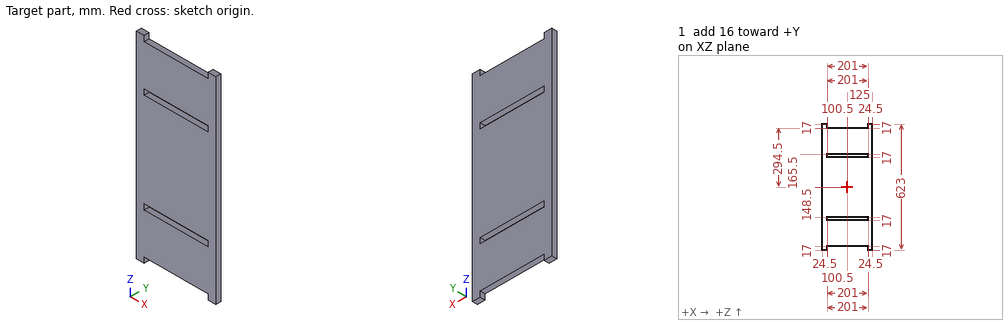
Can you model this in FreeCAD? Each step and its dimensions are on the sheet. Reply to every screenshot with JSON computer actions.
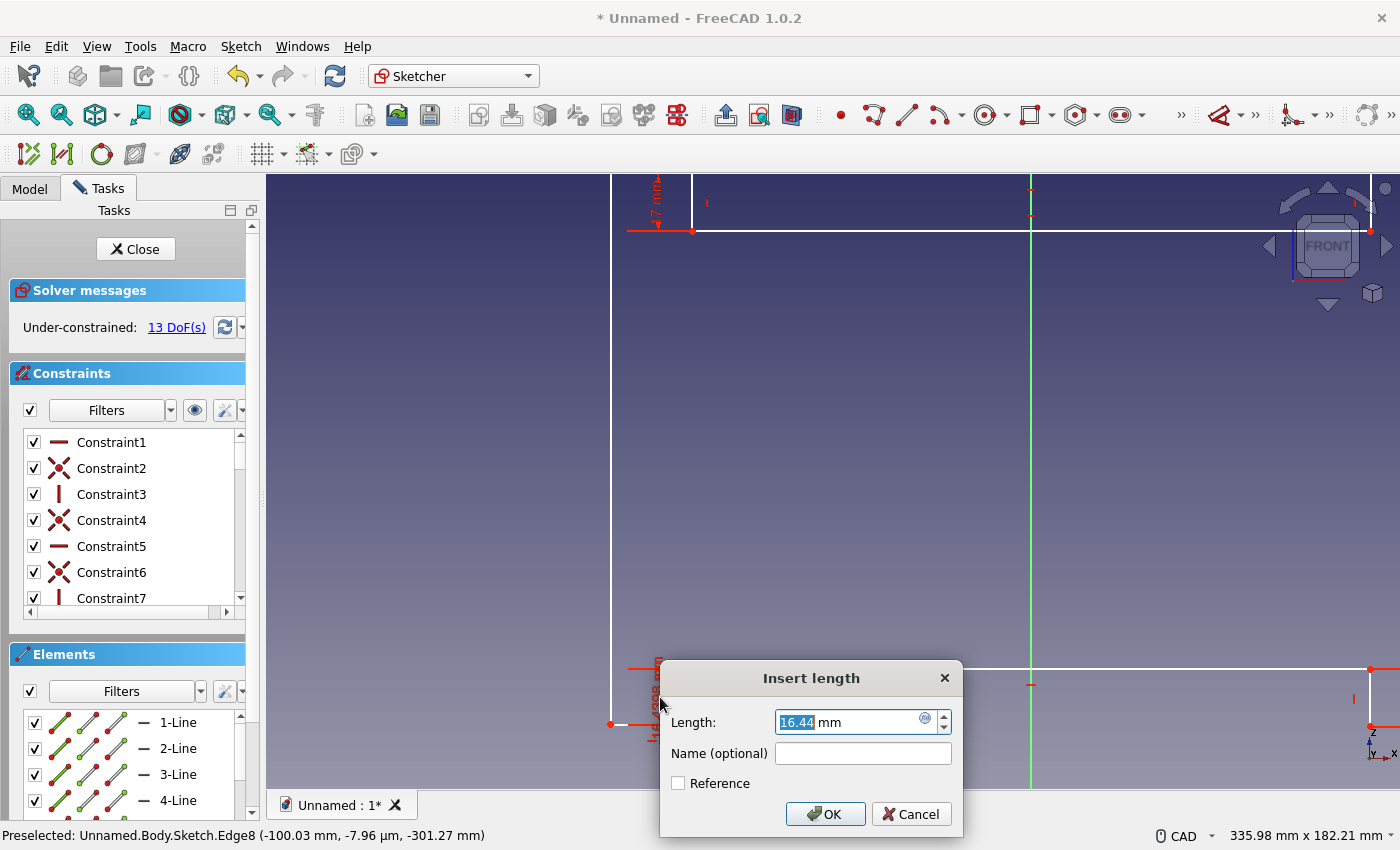
{"action": "type", "text": "17"}
{"action": "key", "text": "Return"}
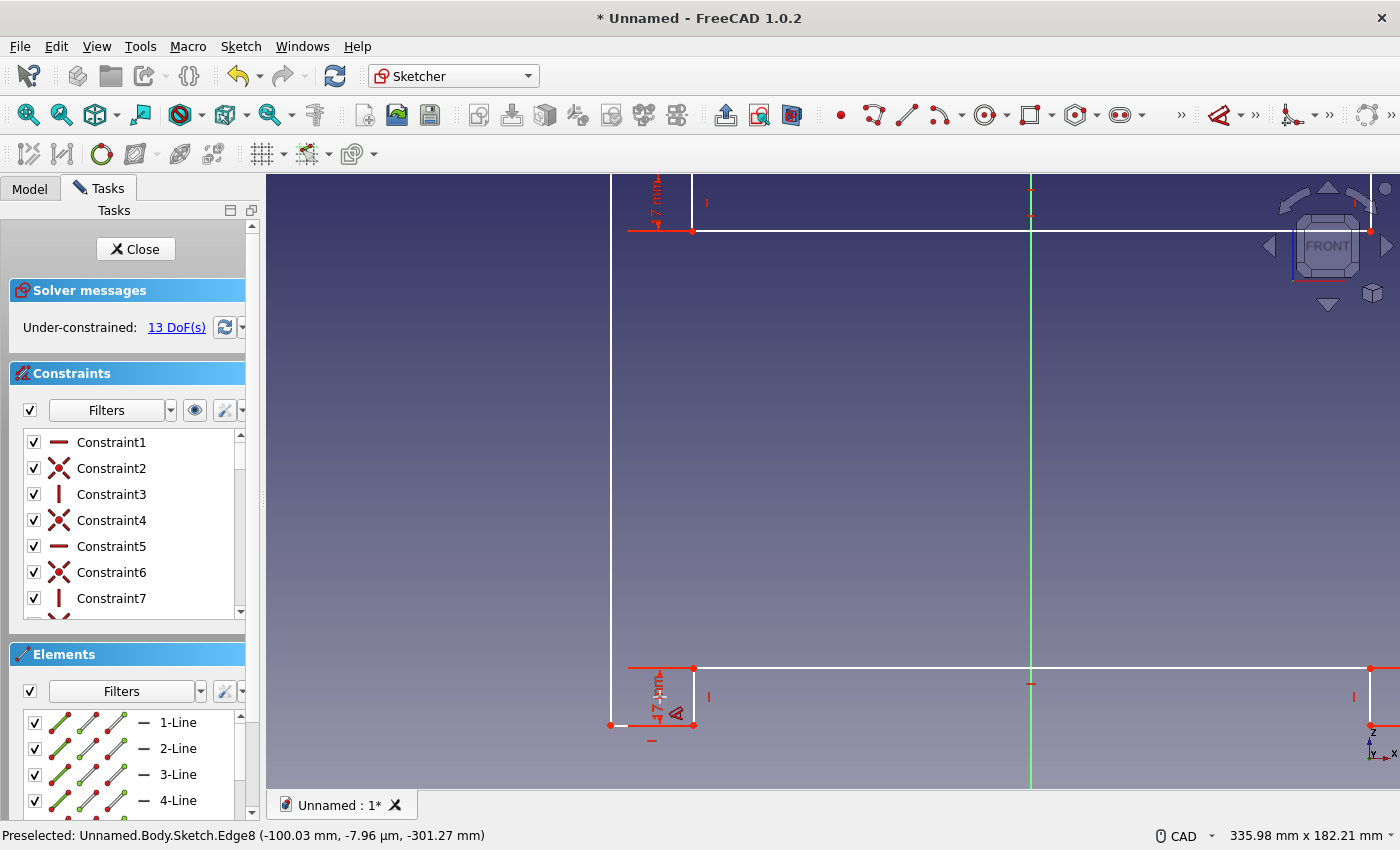
{"action": "scroll", "coordinate": [697, 687], "scroll_direction": "down", "scroll_amount": 8}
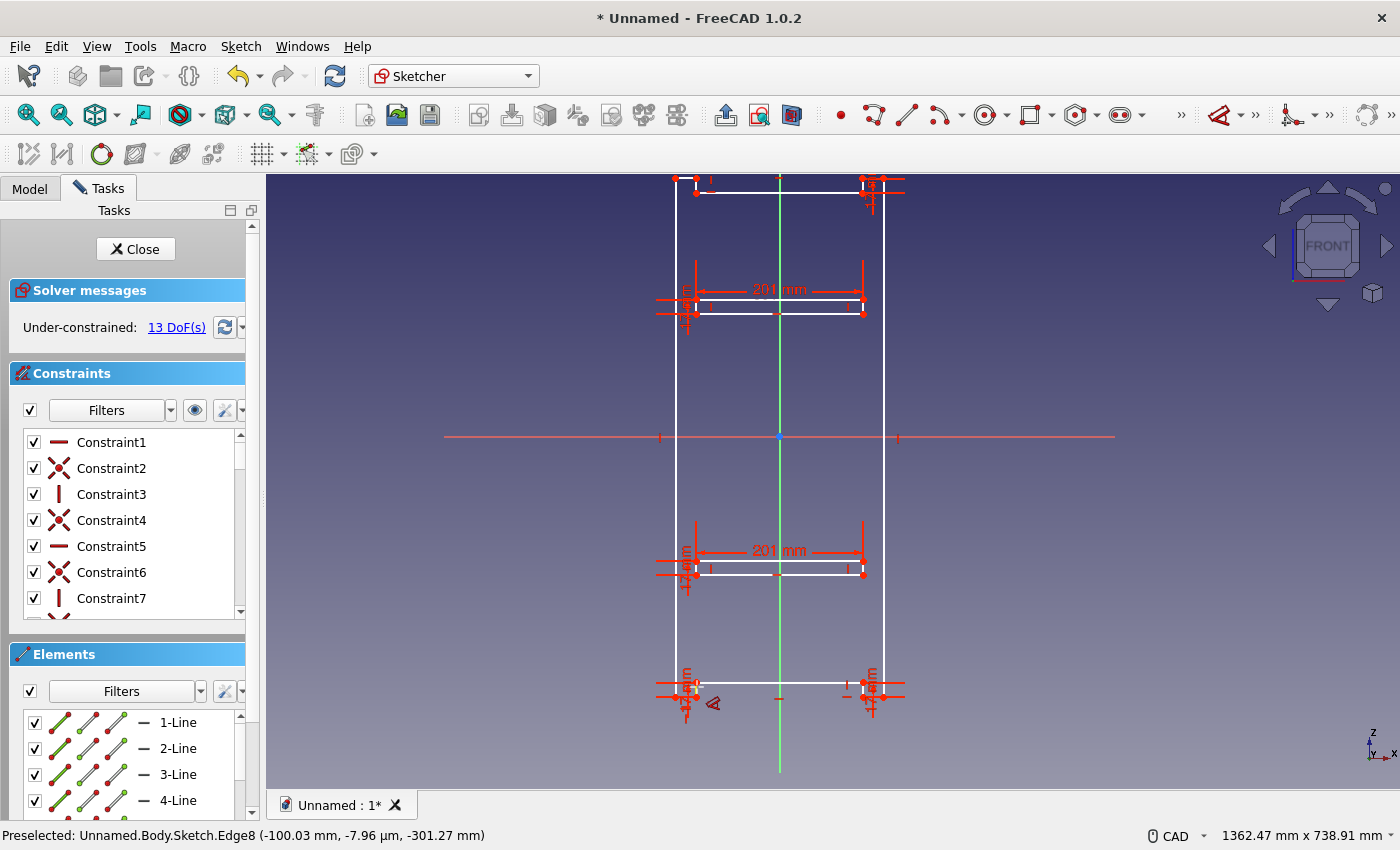
{"action": "scroll", "coordinate": [696, 274], "scroll_direction": "up", "scroll_amount": 7}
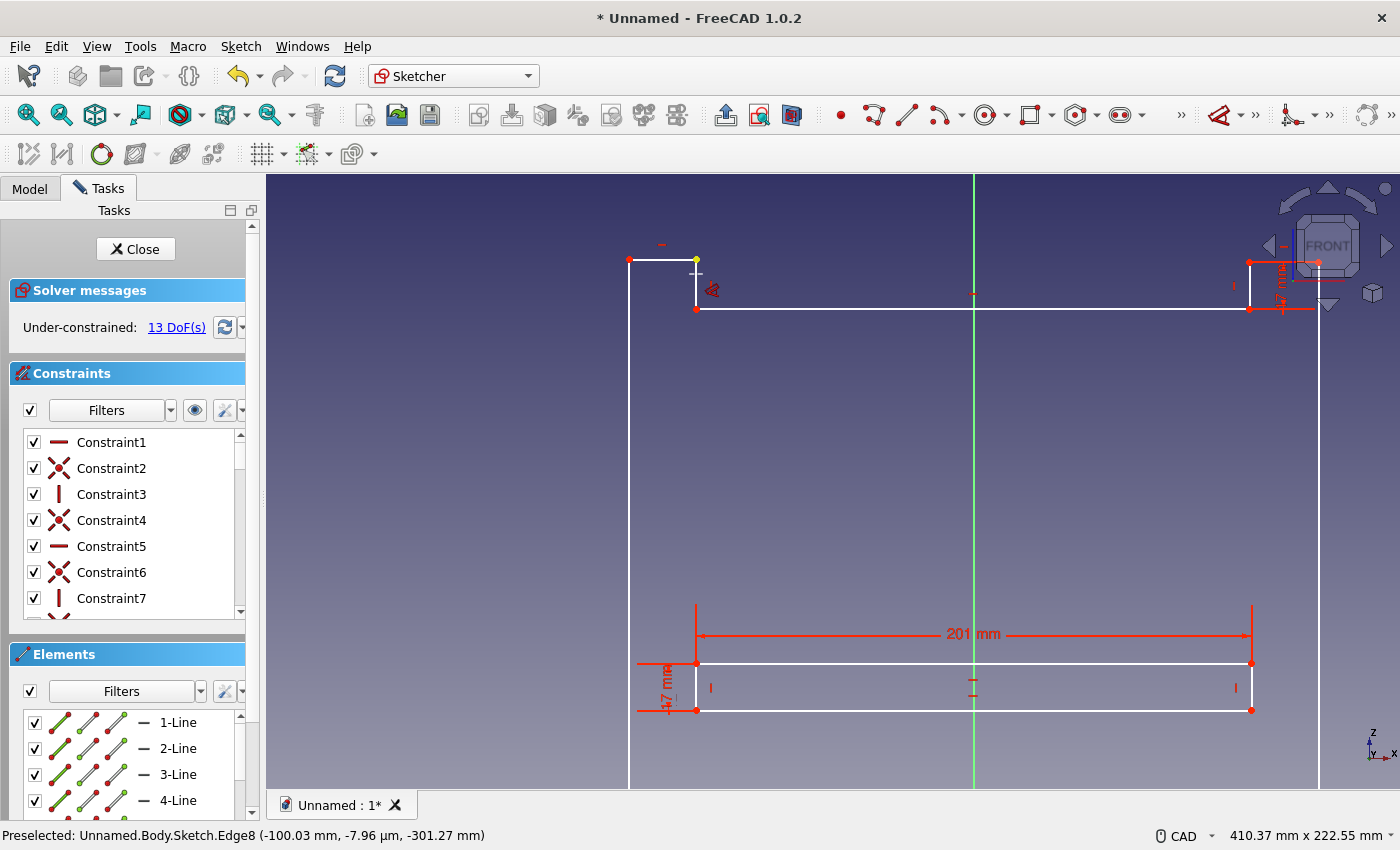
{"action": "left_click", "coordinate": [696, 275]}
{"action": "left_click", "coordinate": [662, 285]}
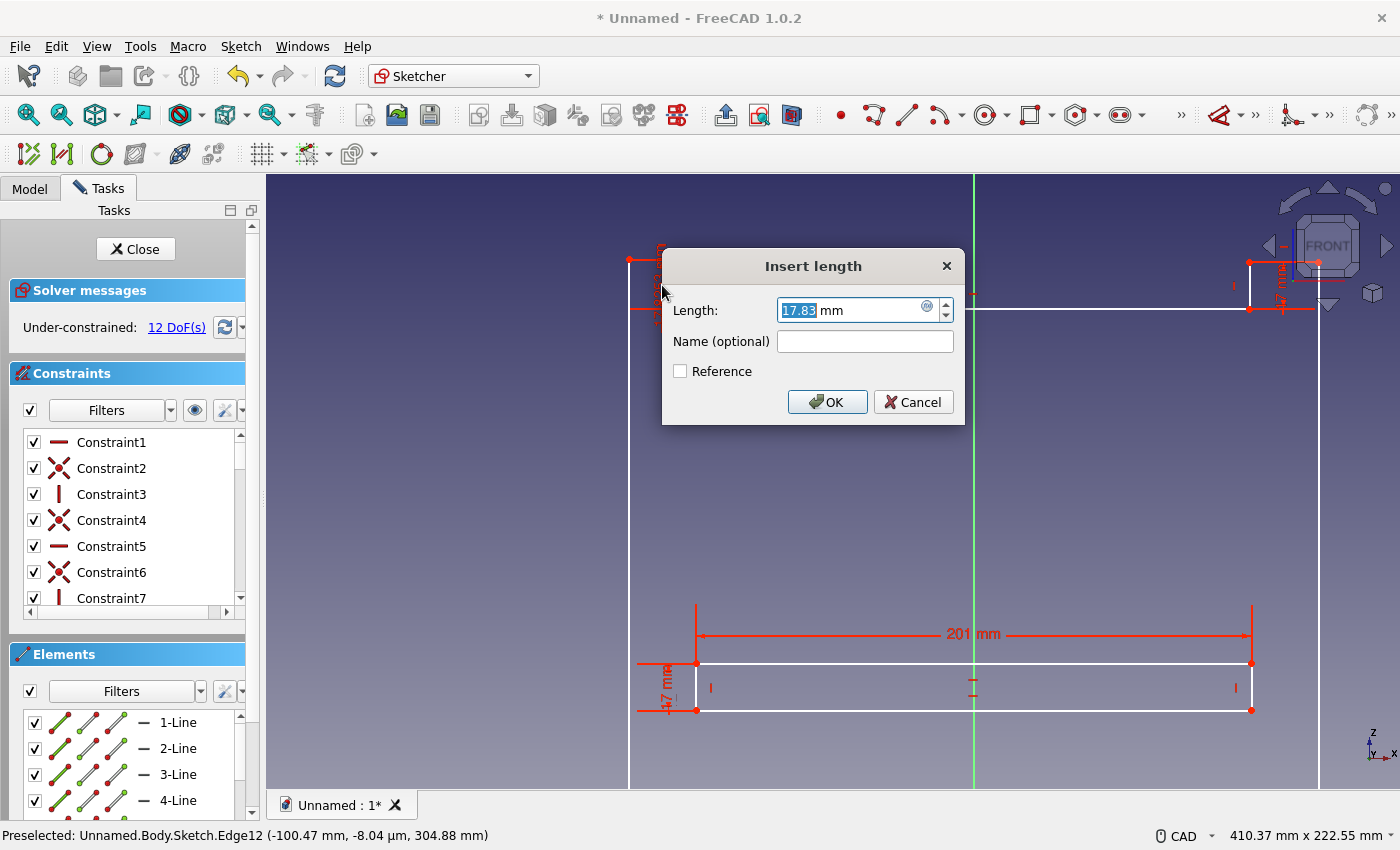
{"action": "type", "text": "17"}
{"action": "key", "text": "Return"}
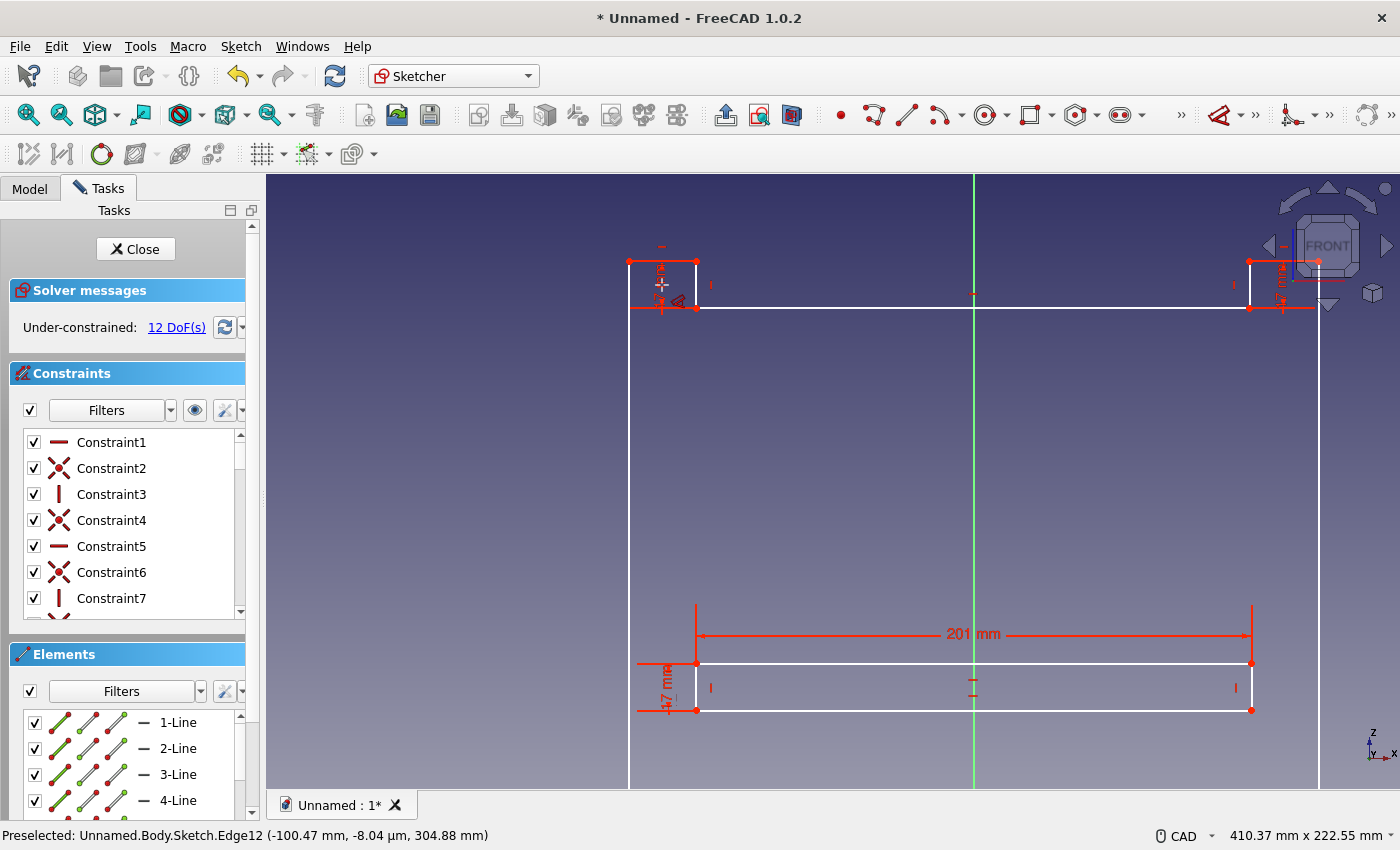
{"action": "scroll", "coordinate": [696, 273], "scroll_direction": "down", "scroll_amount": 7}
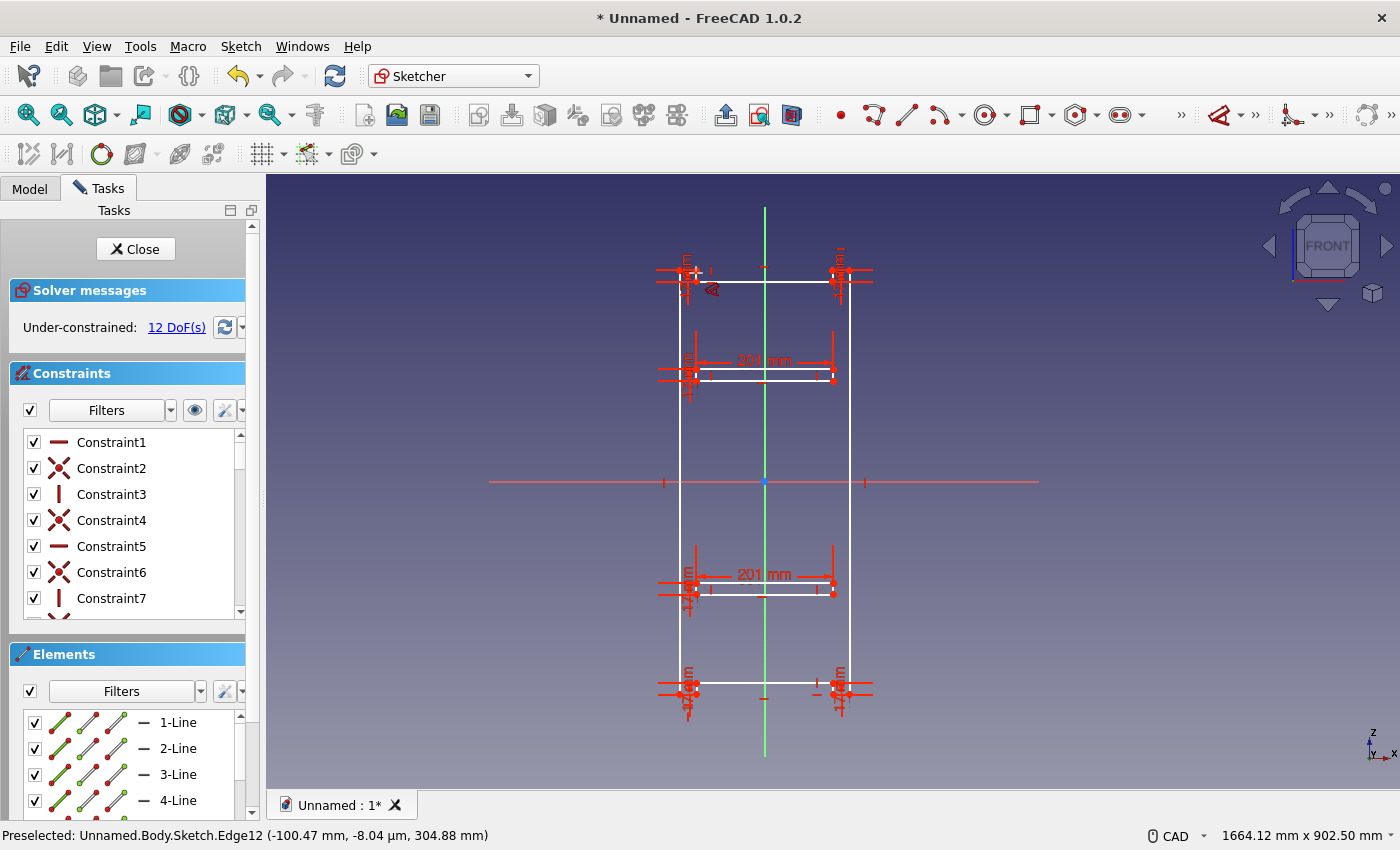
{"action": "left_click", "coordinate": [737, 282]}
{"action": "left_click", "coordinate": [733, 248]}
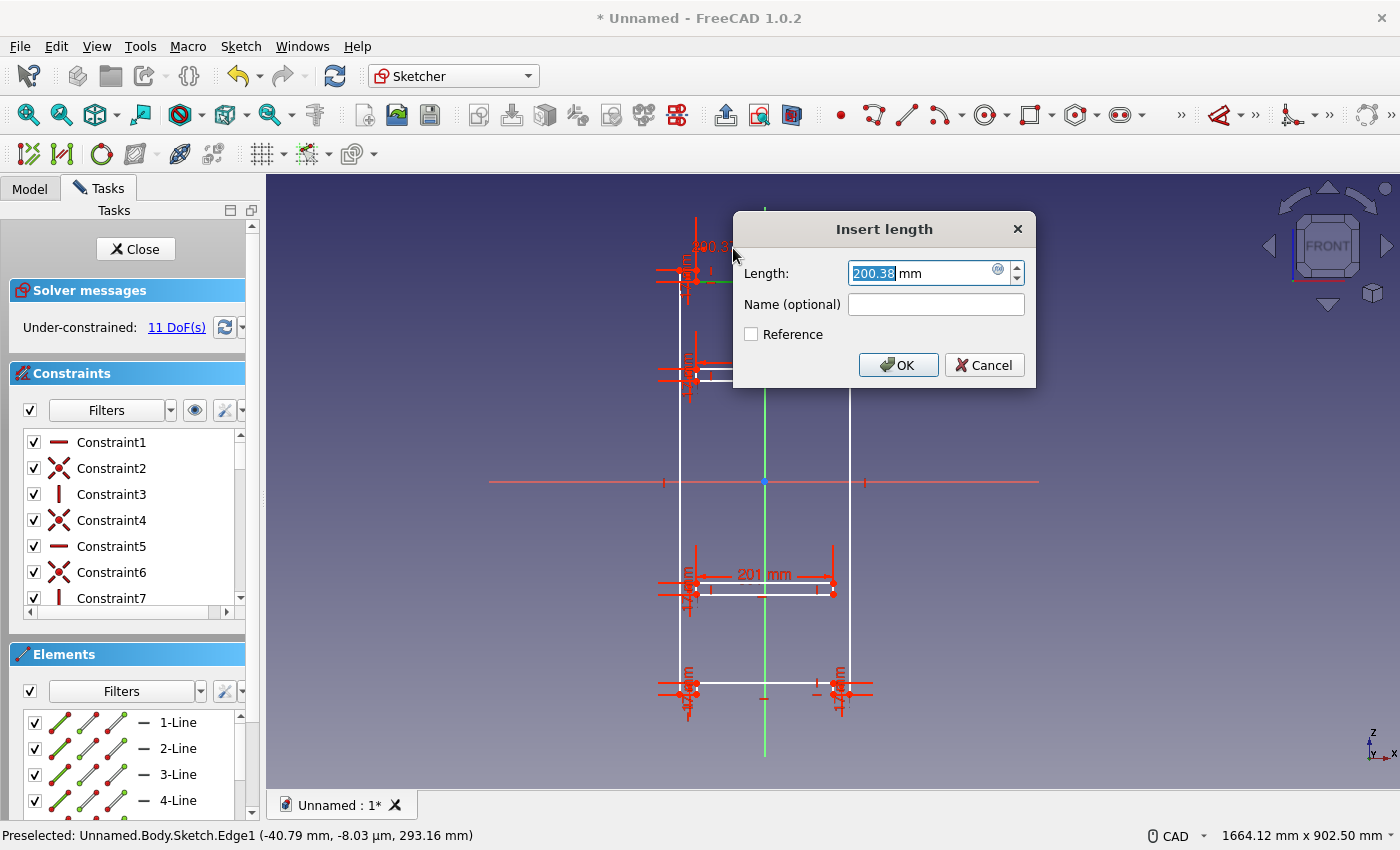
{"action": "type", "text": "201"}
{"action": "key", "text": "Return"}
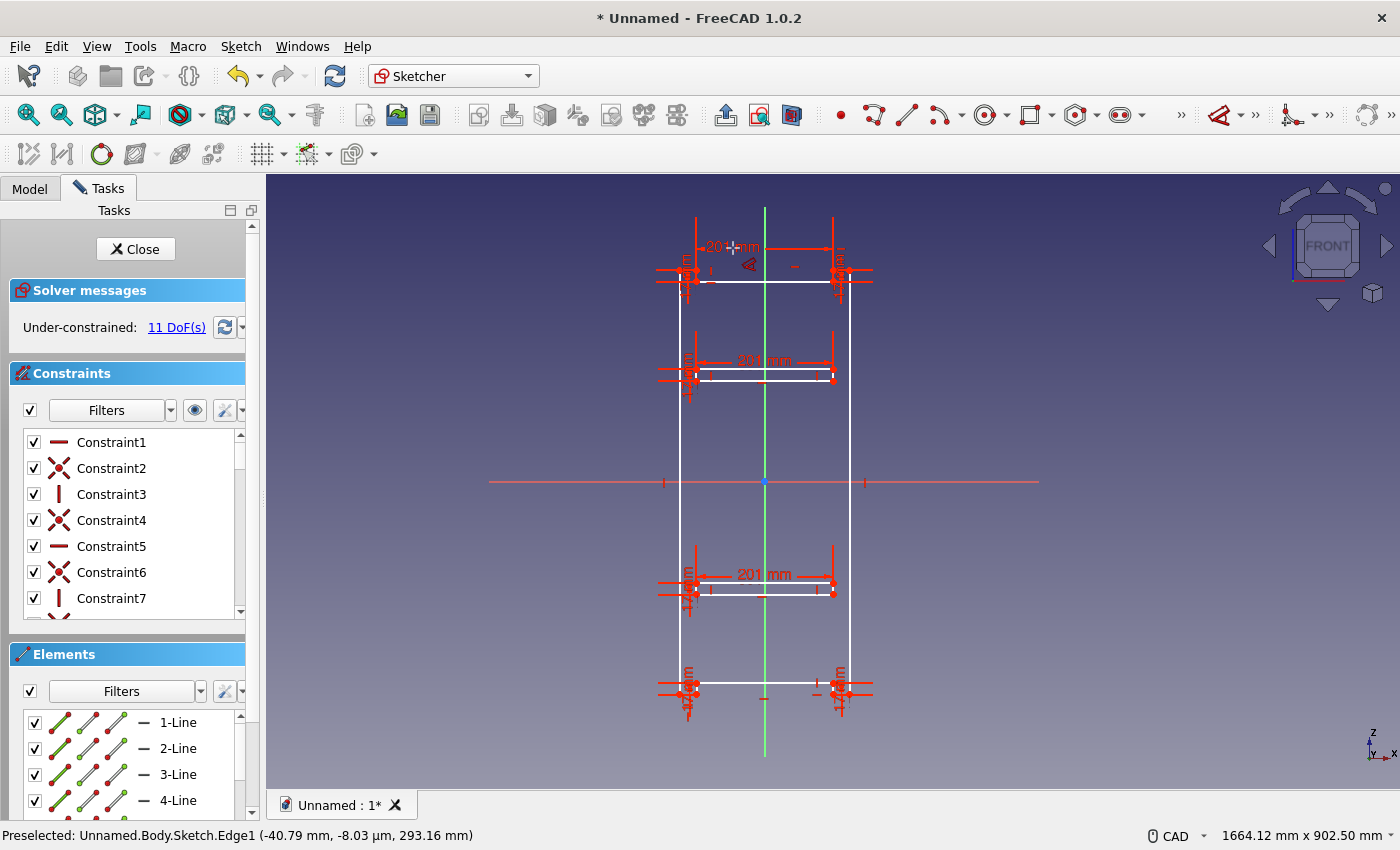
{"action": "left_click", "coordinate": [850, 398]}
{"action": "left_click", "coordinate": [884, 385]}